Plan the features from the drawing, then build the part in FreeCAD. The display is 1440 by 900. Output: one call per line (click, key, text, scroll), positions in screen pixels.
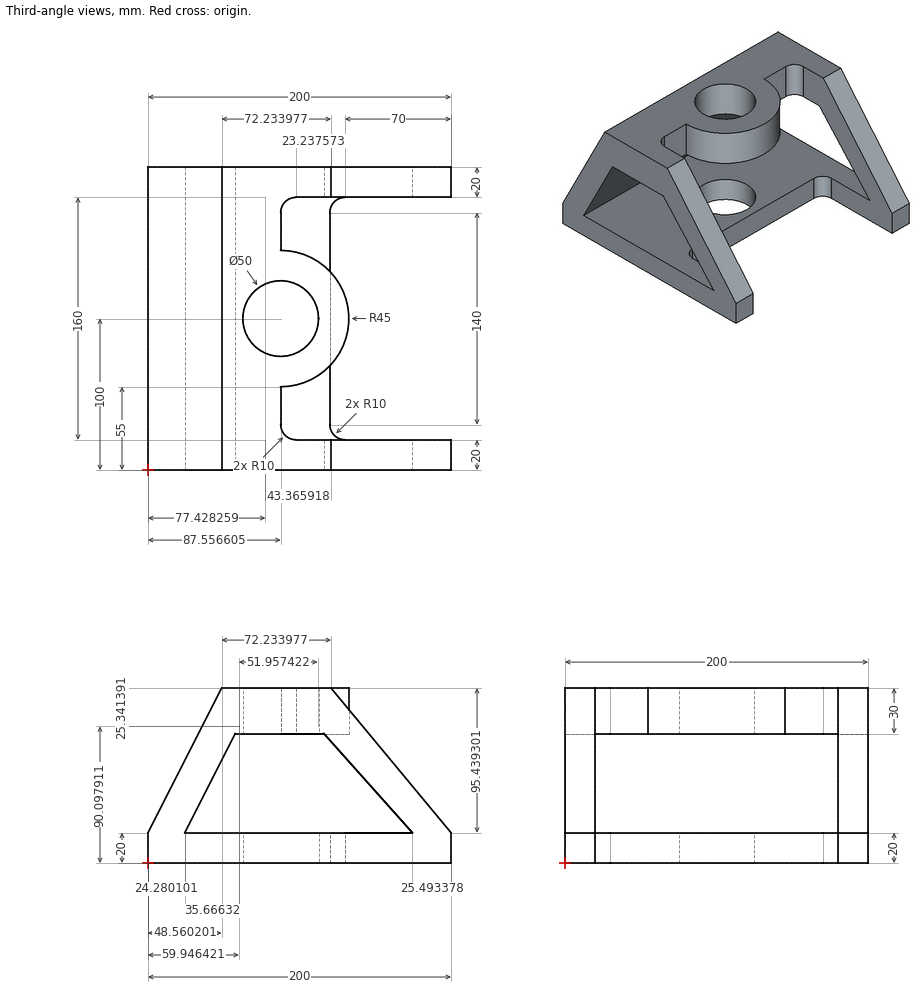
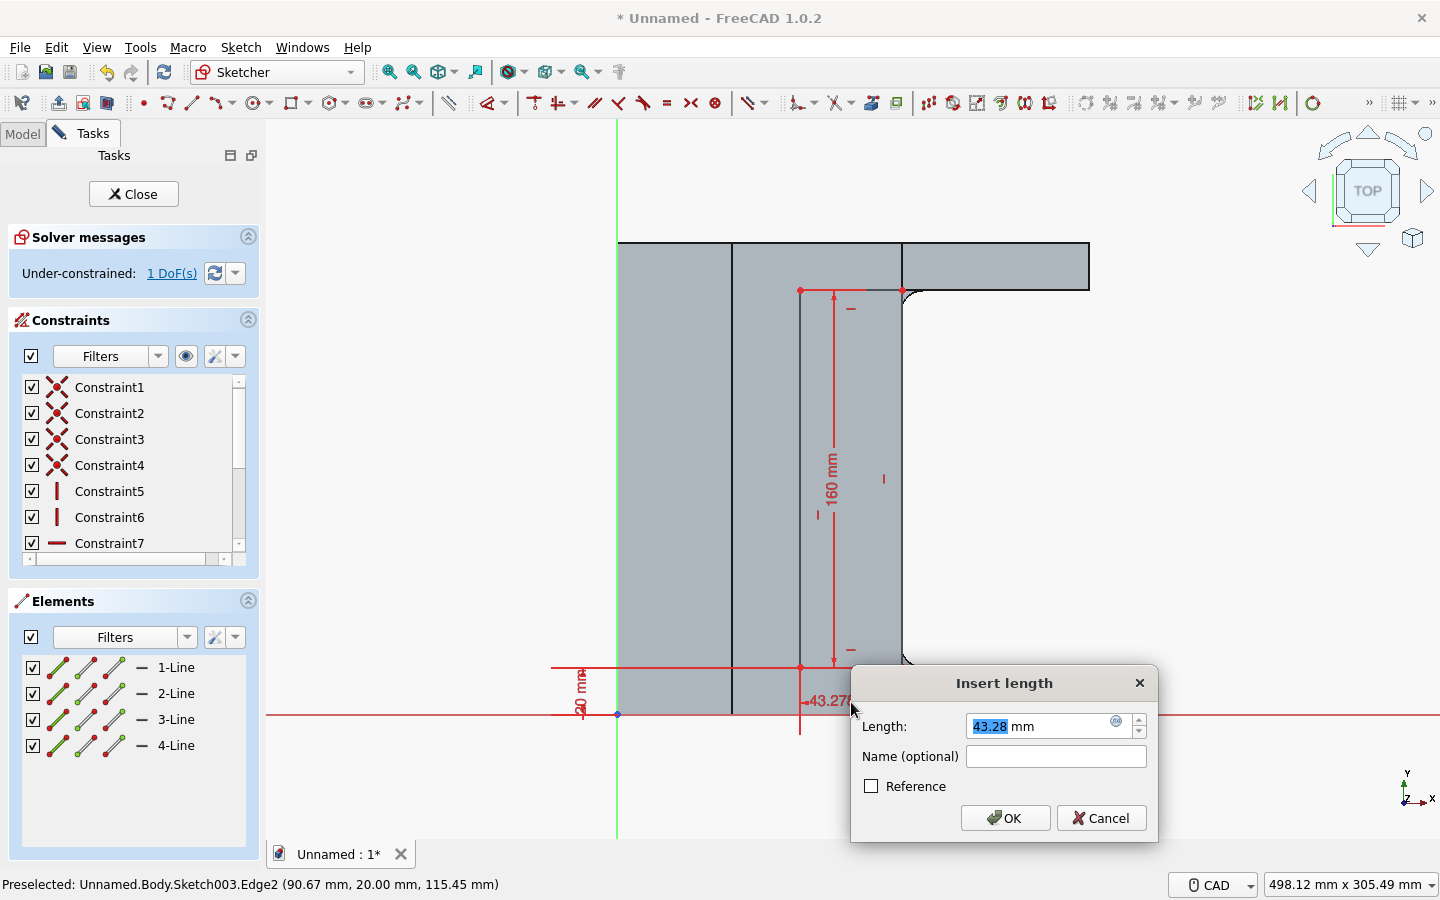
text(43.365918)
key(Return)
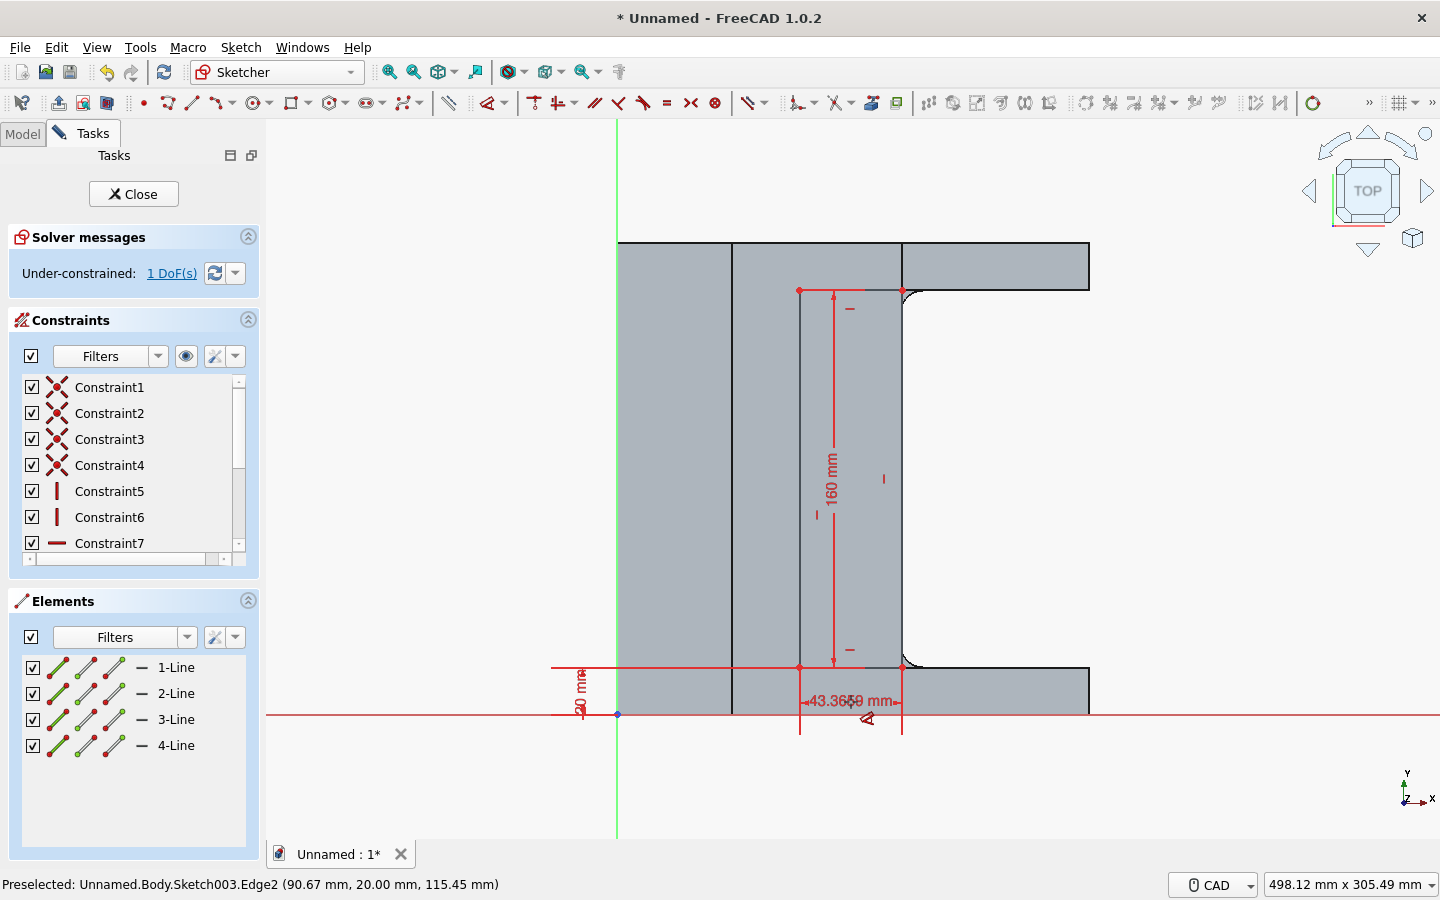
click(800, 290)
click(709, 749)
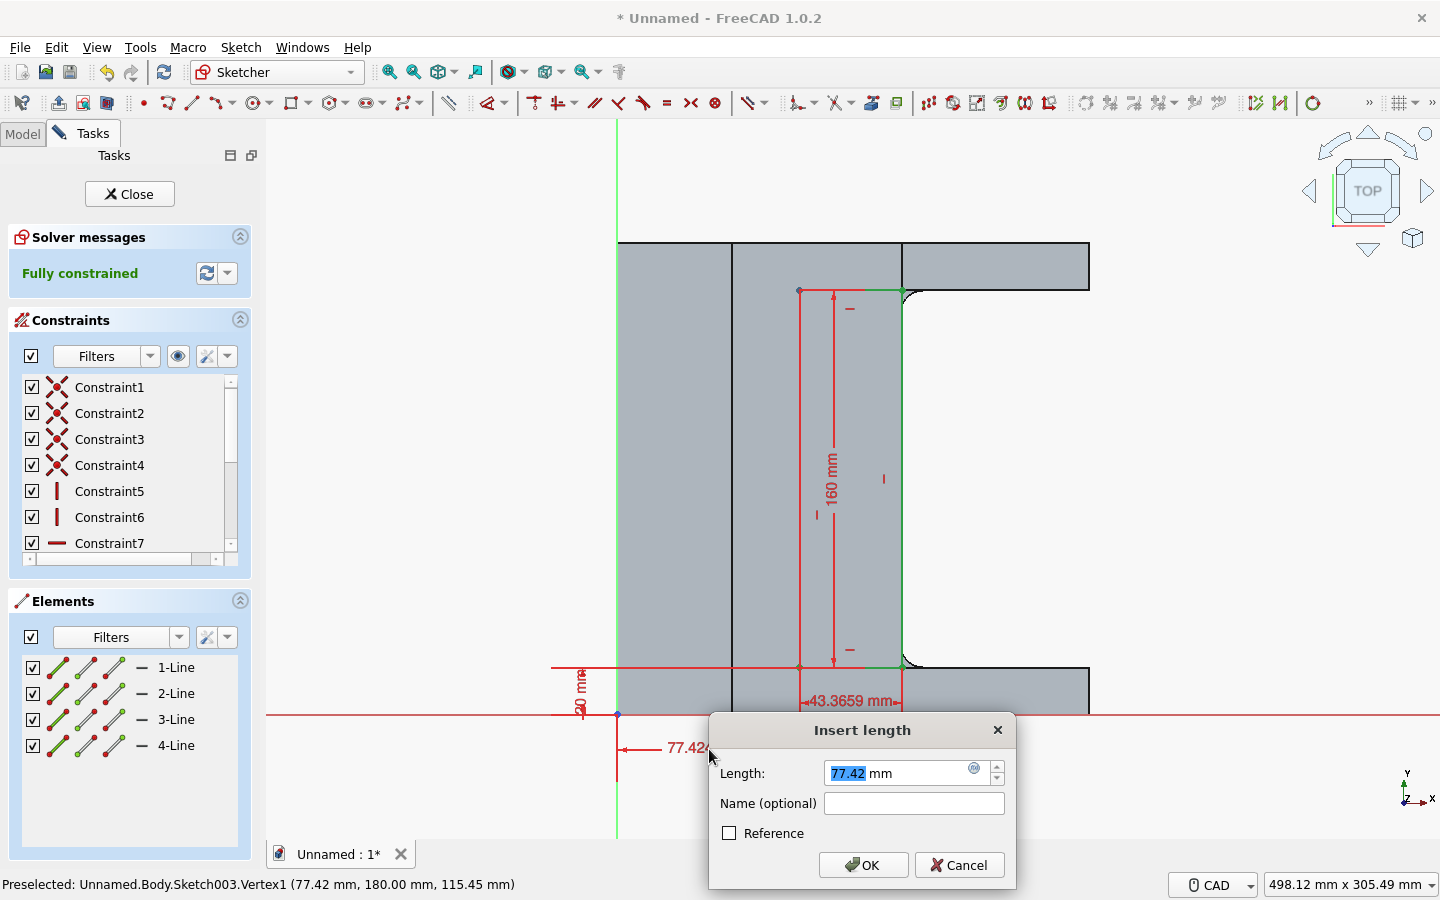
text(77.428259)
key(Return)
key(Escape)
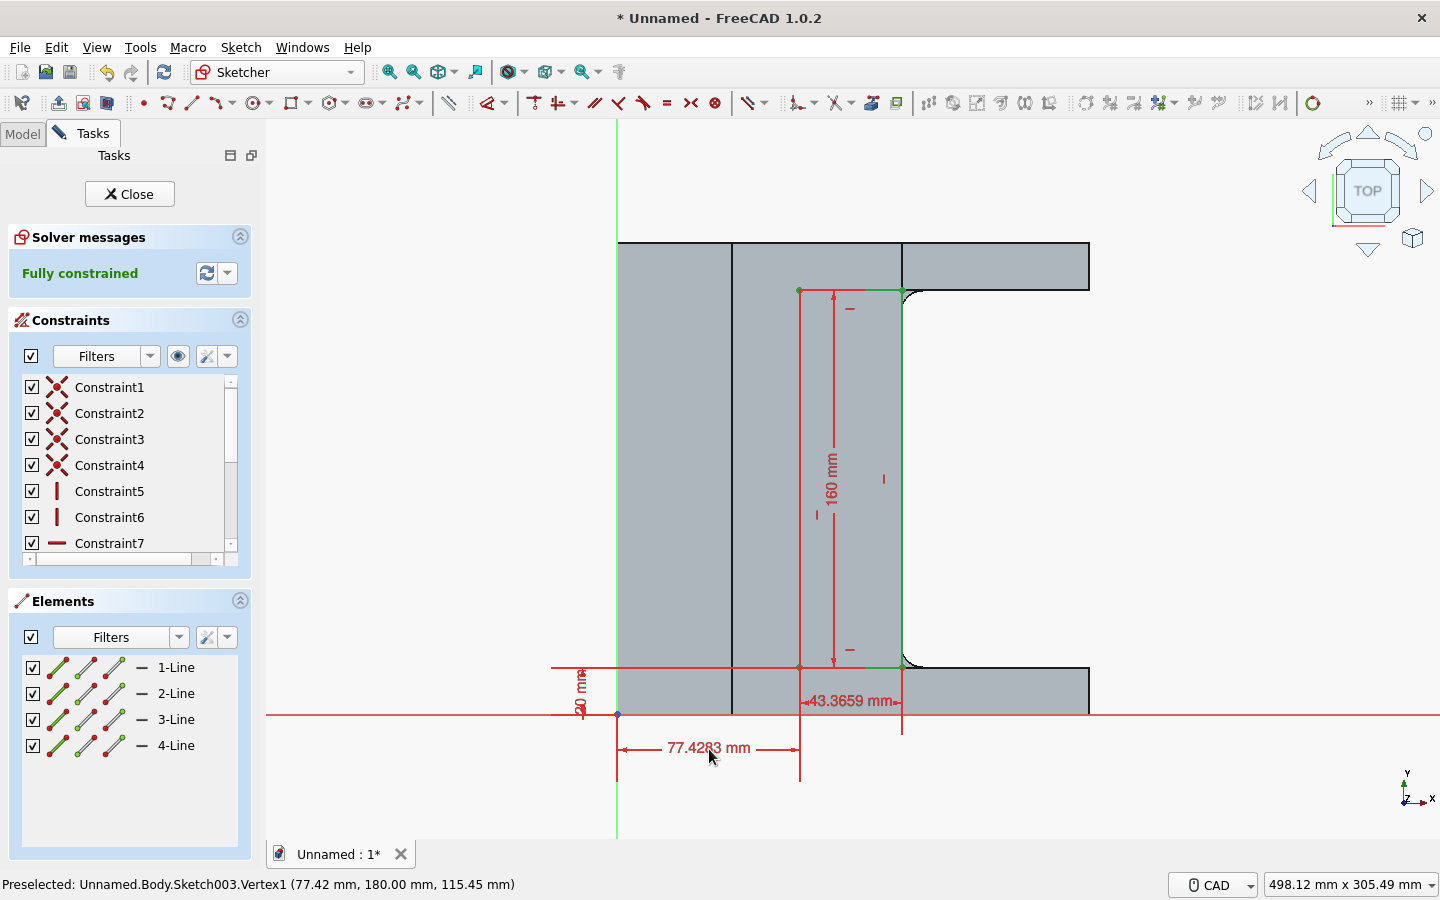
click(130, 194)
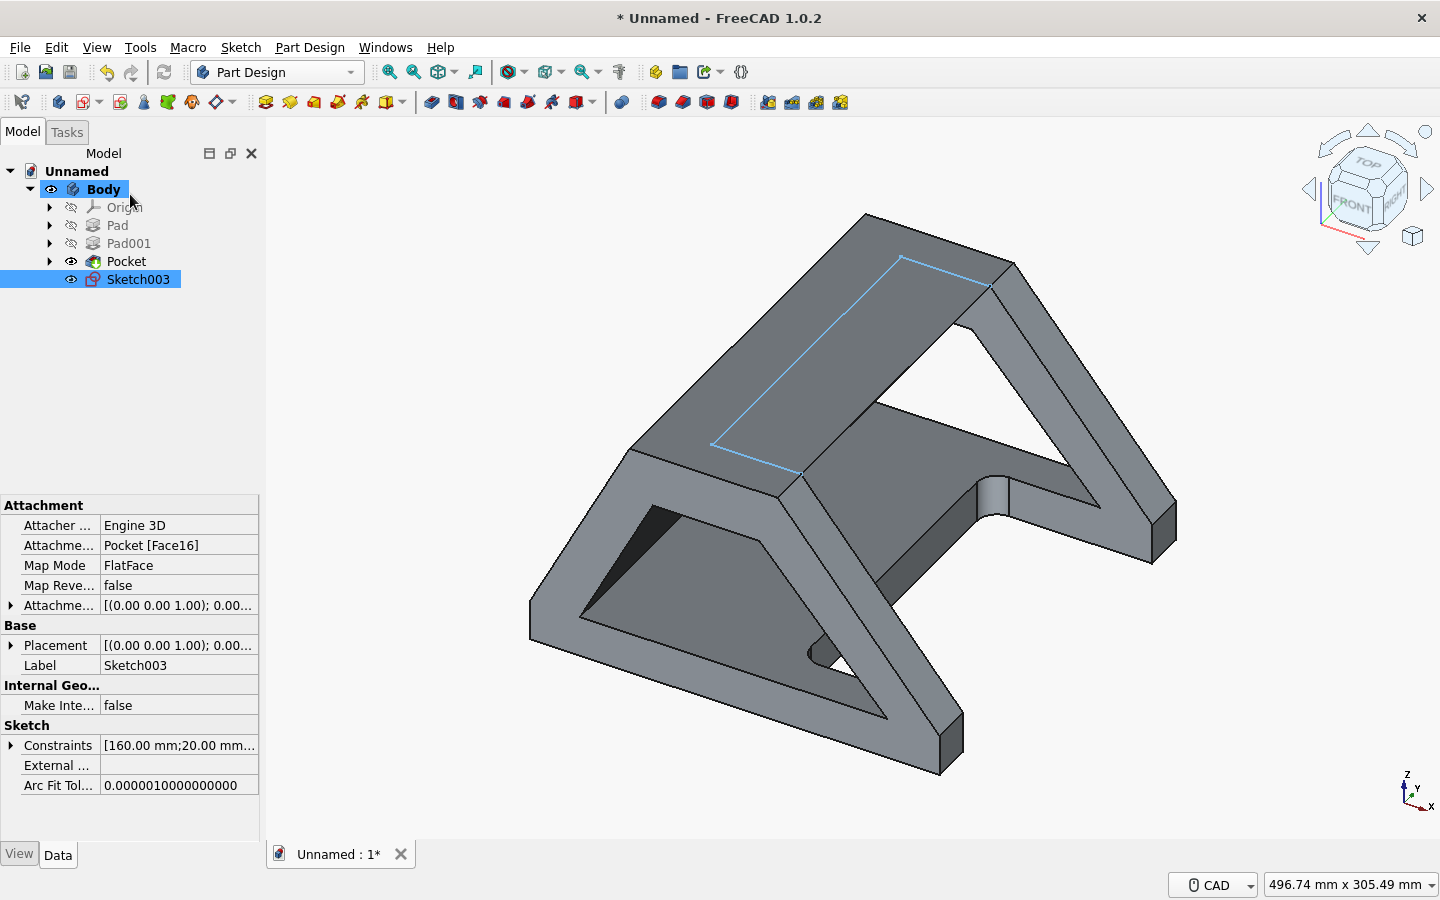
click(432, 102)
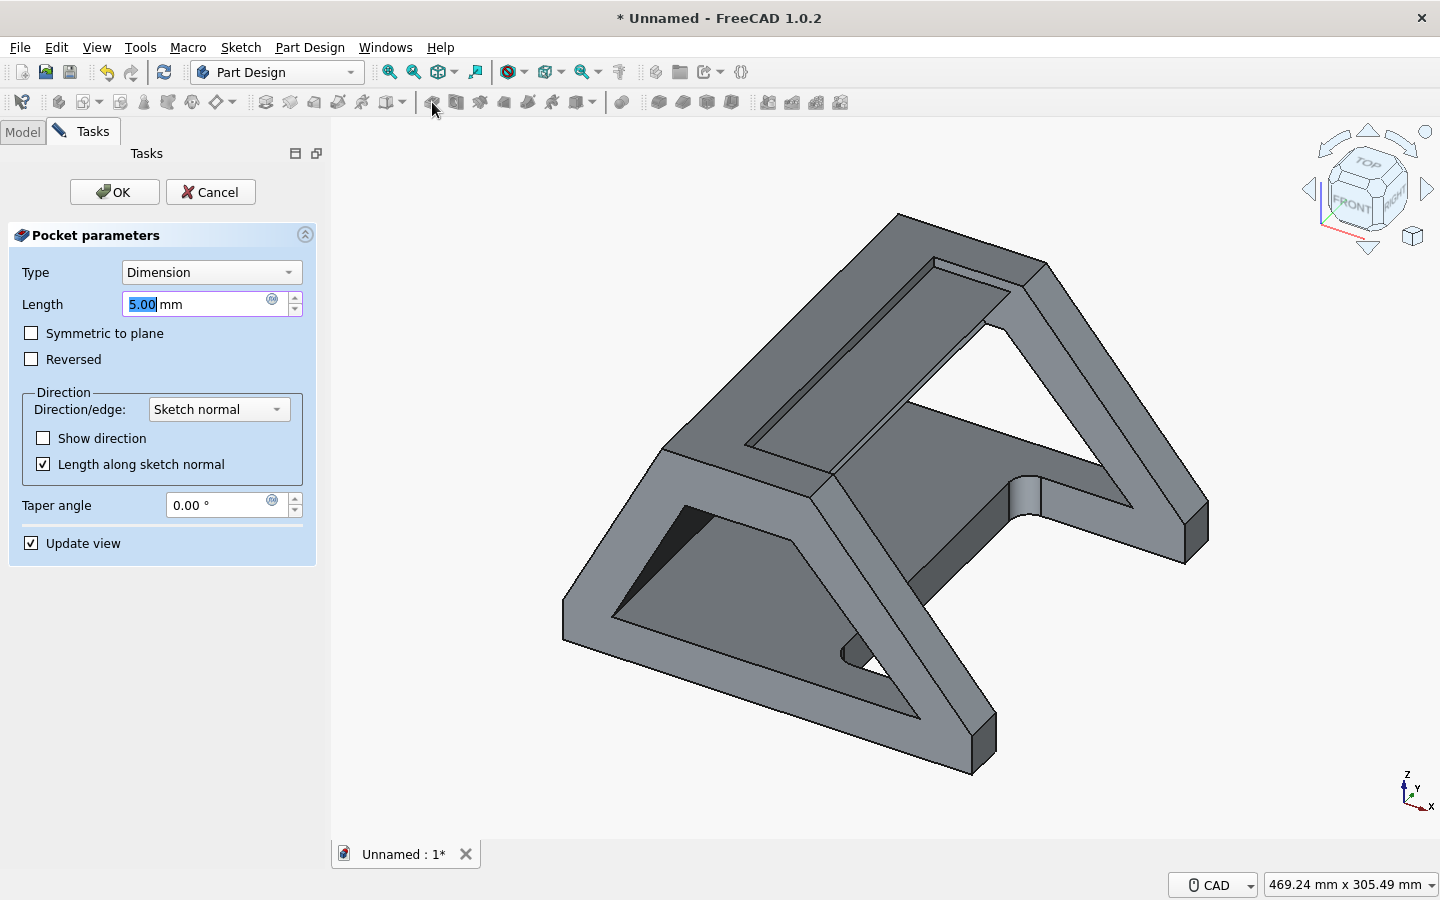
text(30)
key(Tab)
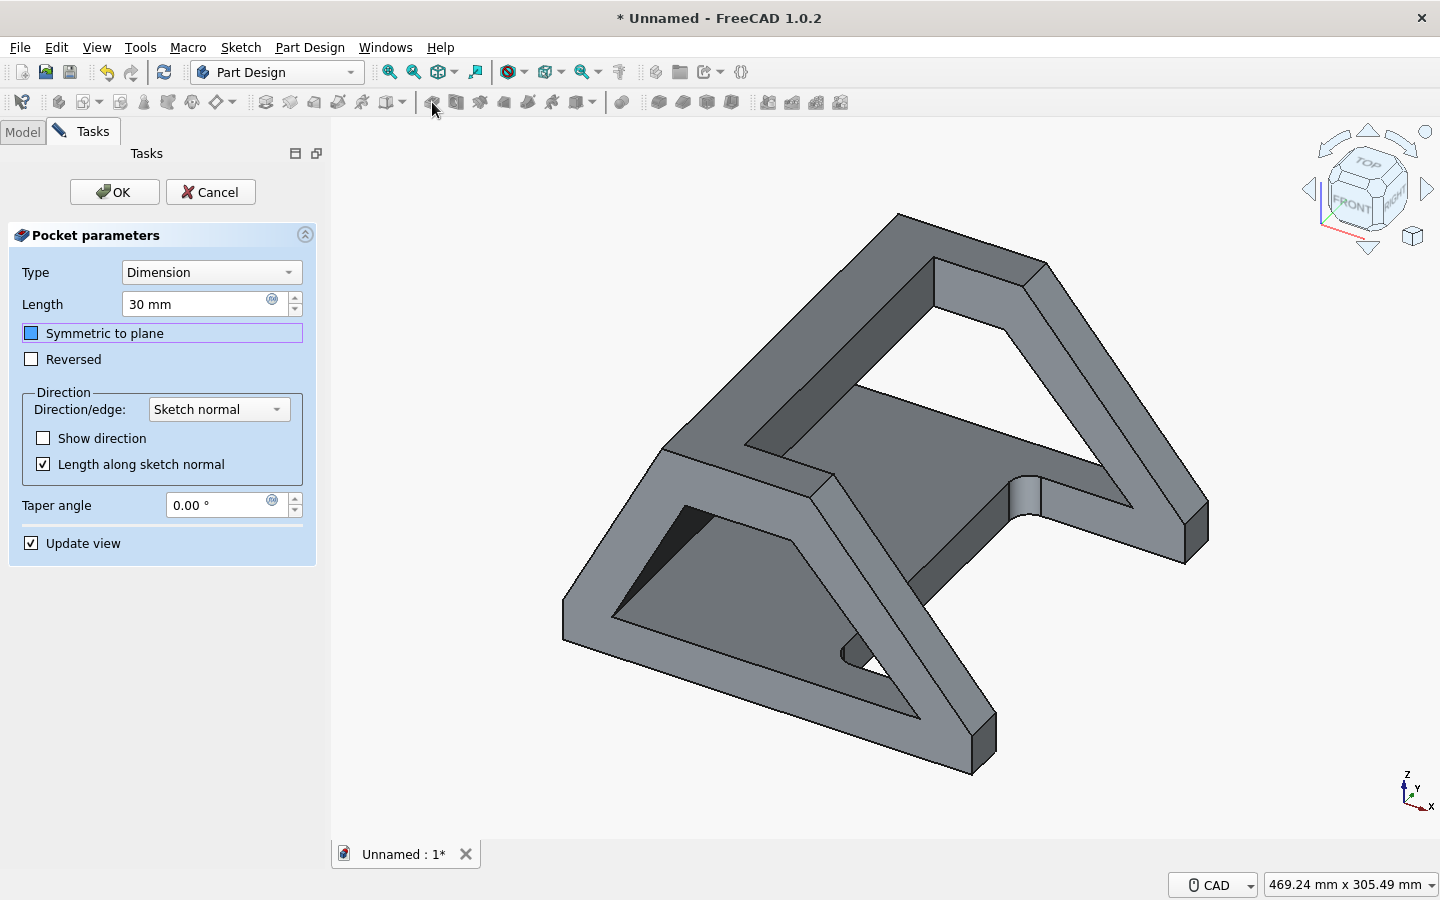
click(115, 192)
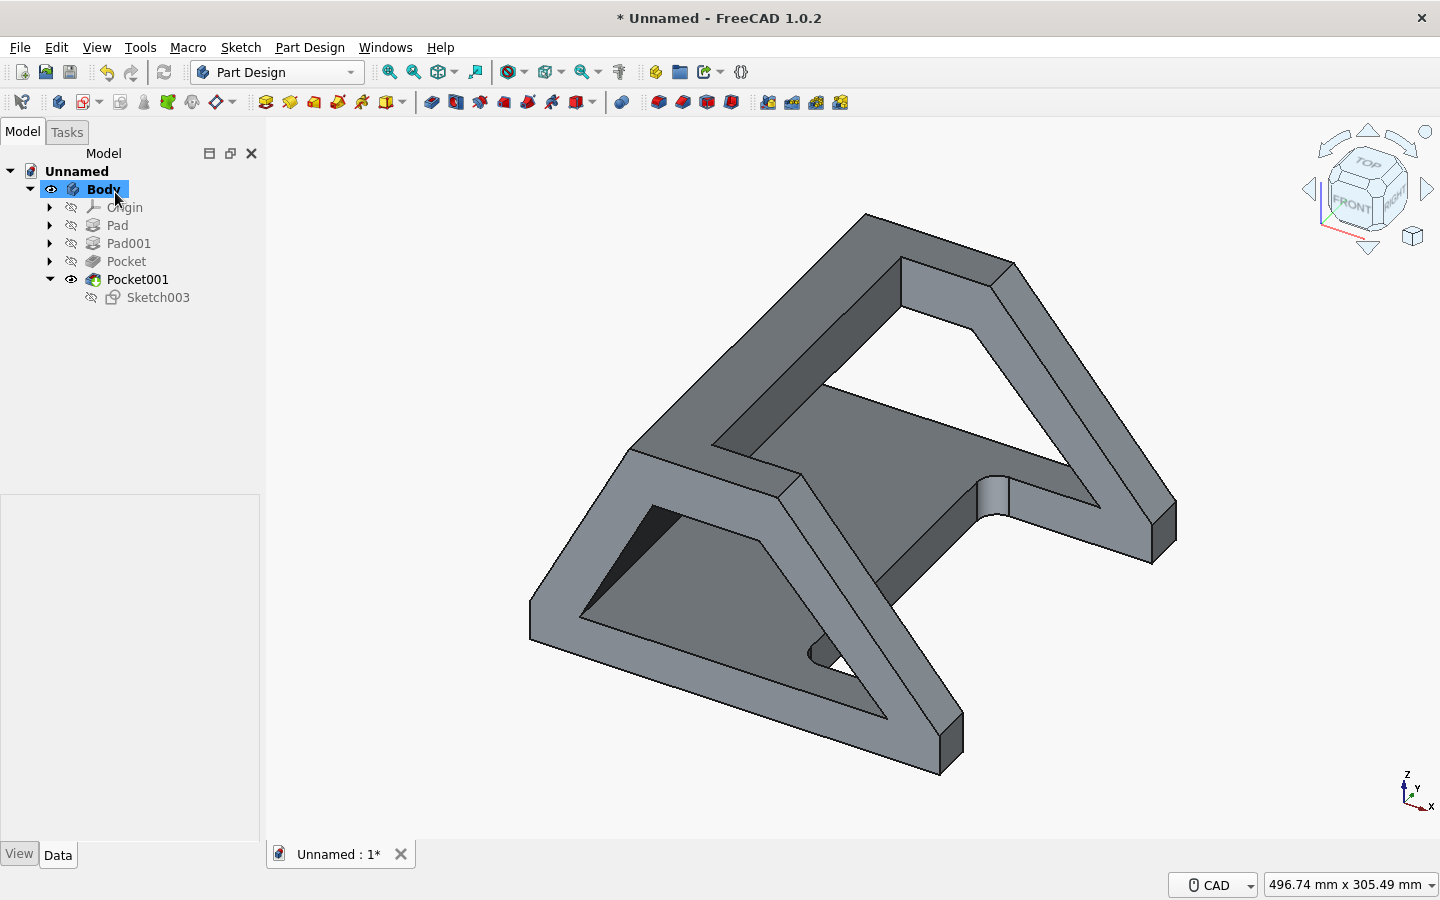
click(84, 102)